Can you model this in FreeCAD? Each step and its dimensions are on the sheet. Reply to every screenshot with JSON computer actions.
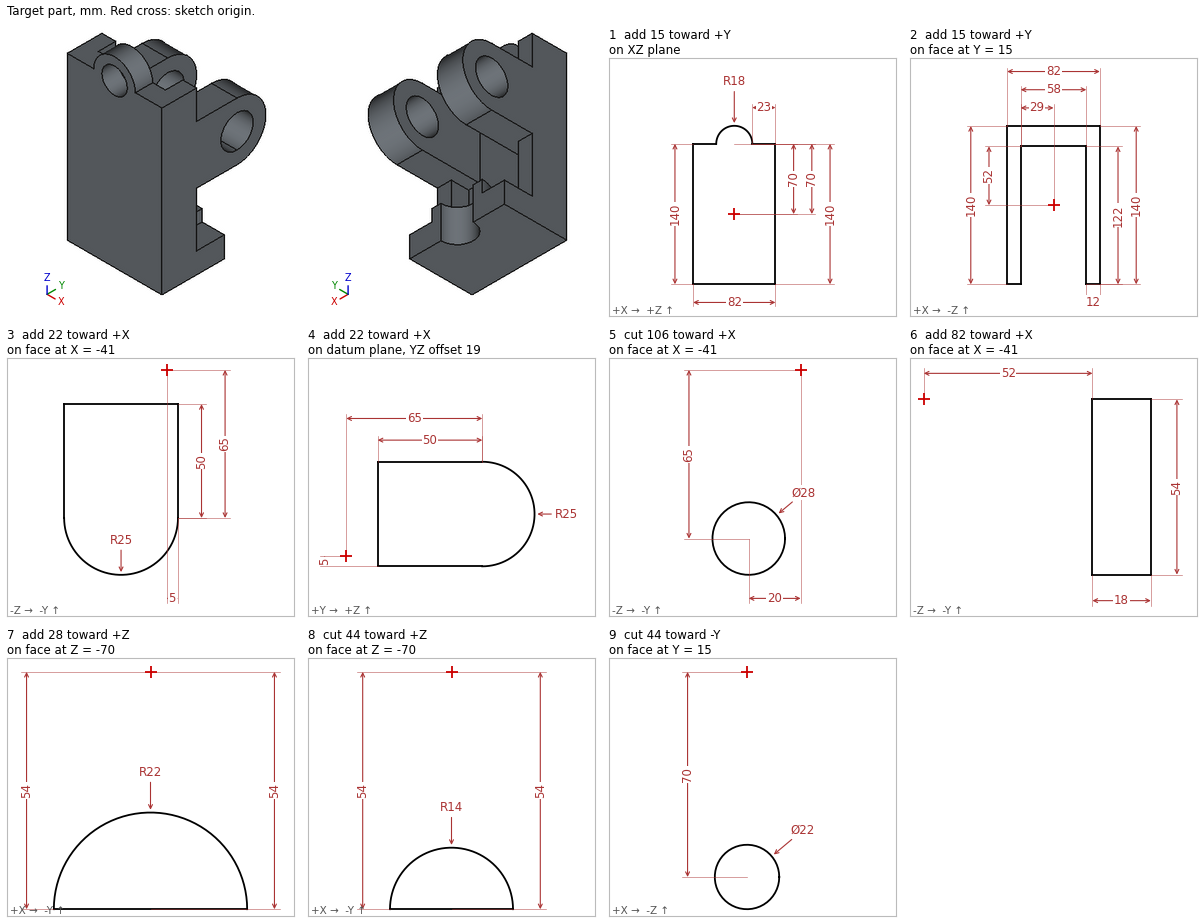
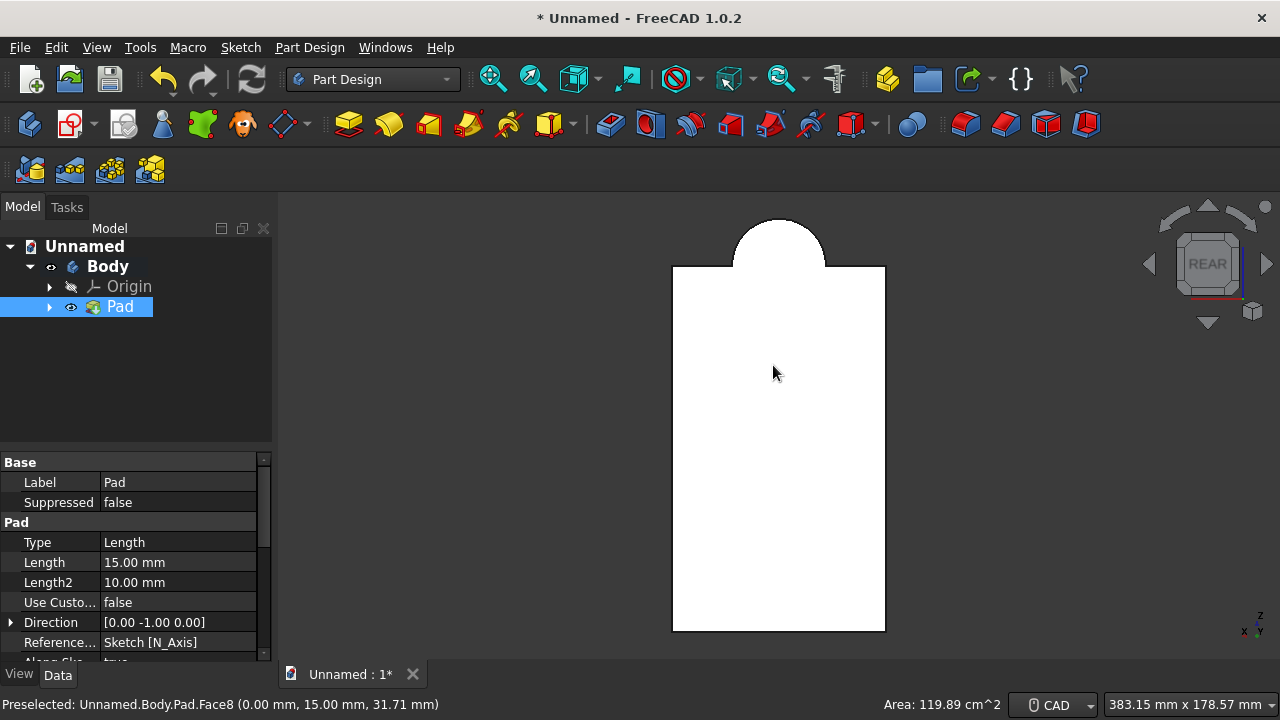
{"action": "left_click", "coordinate": [70, 124]}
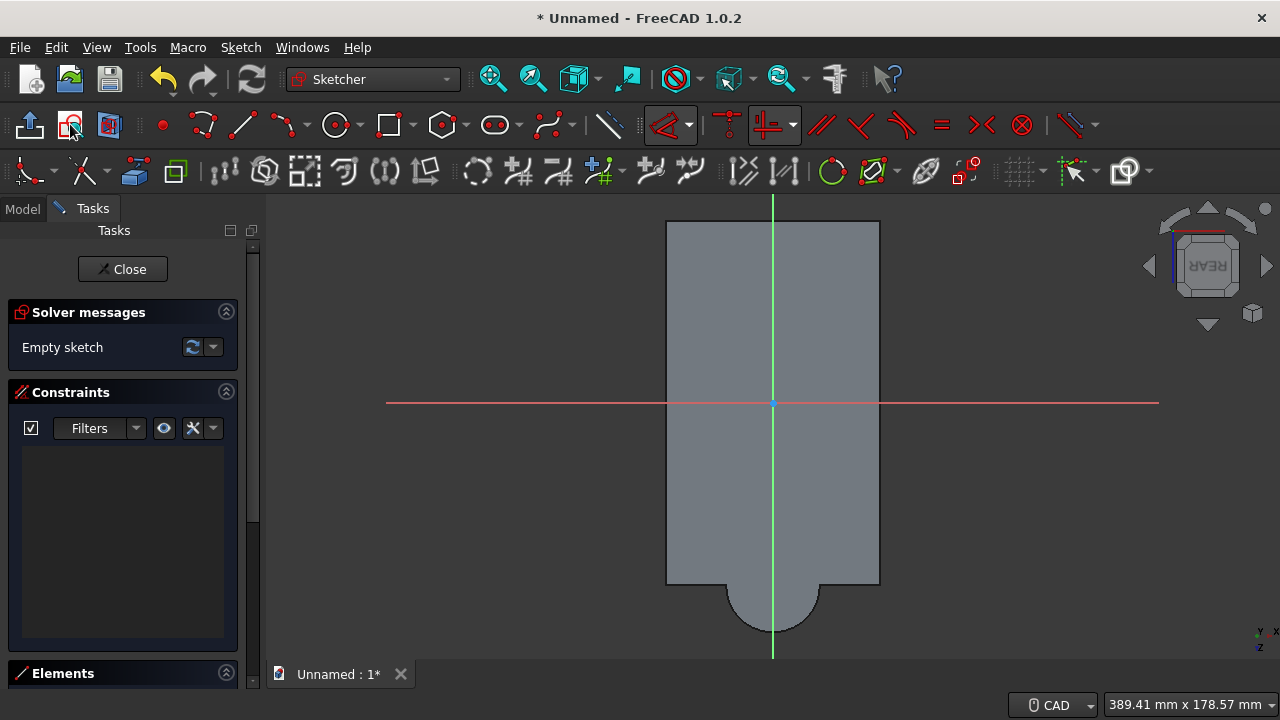
{"action": "scroll", "coordinate": [395, 532], "scroll_direction": "down", "scroll_amount": 1}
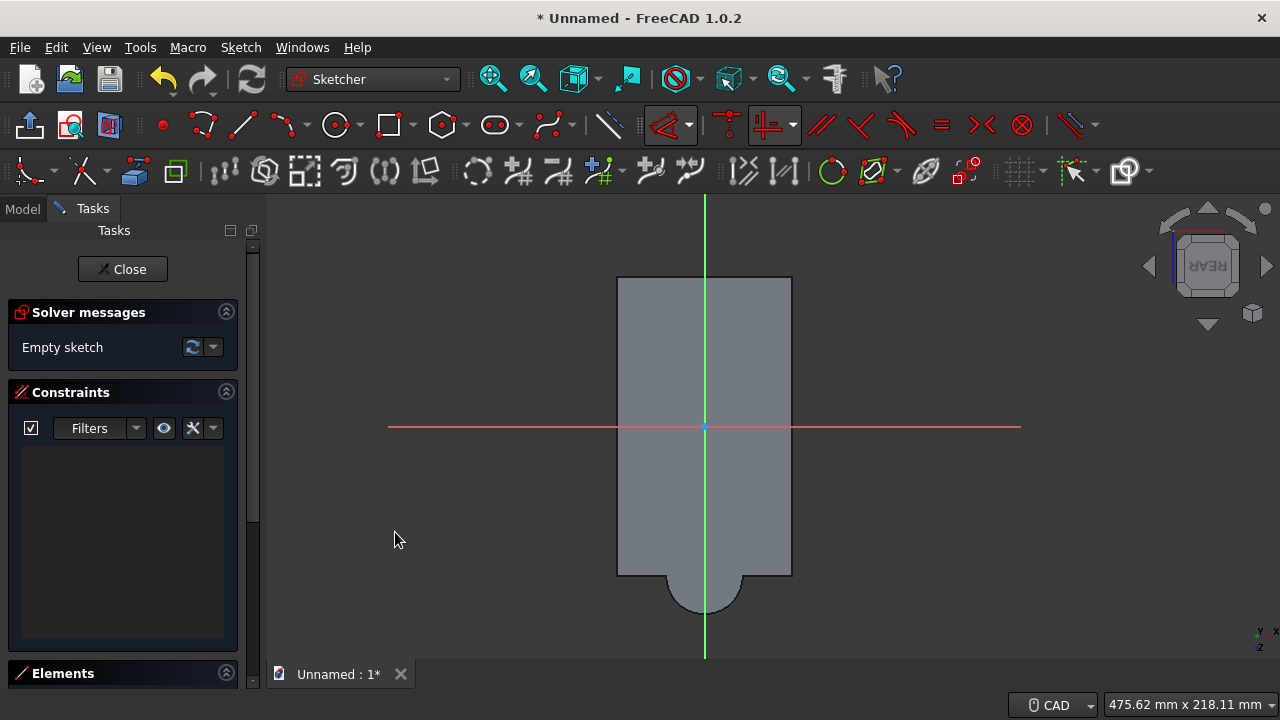
{"action": "key", "text": "g m"}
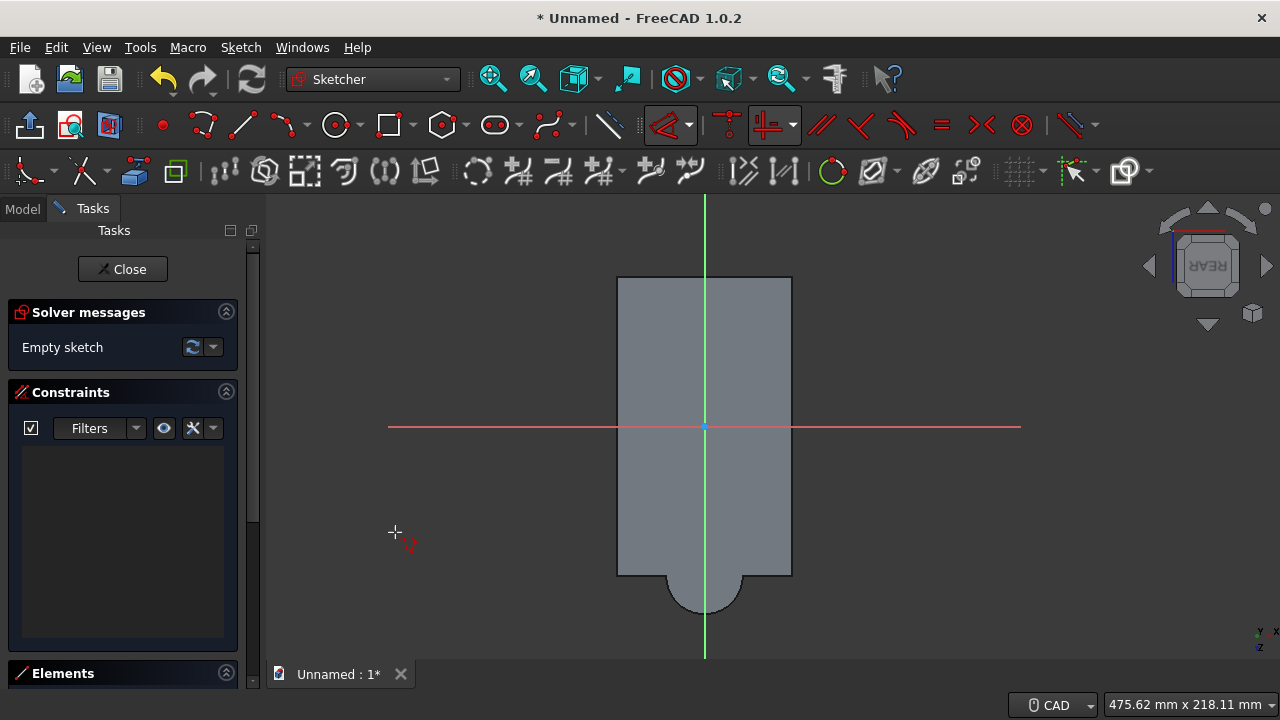
{"action": "left_click", "coordinate": [643, 316]}
{"action": "left_click", "coordinate": [766, 316]}
{"action": "left_click", "coordinate": [766, 576]}
{"action": "left_click", "coordinate": [792, 576]}
{"action": "left_click", "coordinate": [792, 277]}
{"action": "left_click", "coordinate": [617, 277]}
{"action": "left_click", "coordinate": [617, 576]}
{"action": "left_click", "coordinate": [643, 576]}
{"action": "left_click", "coordinate": [643, 317]}
{"action": "key", "text": "Escape"}
{"action": "key", "text": "Escape"}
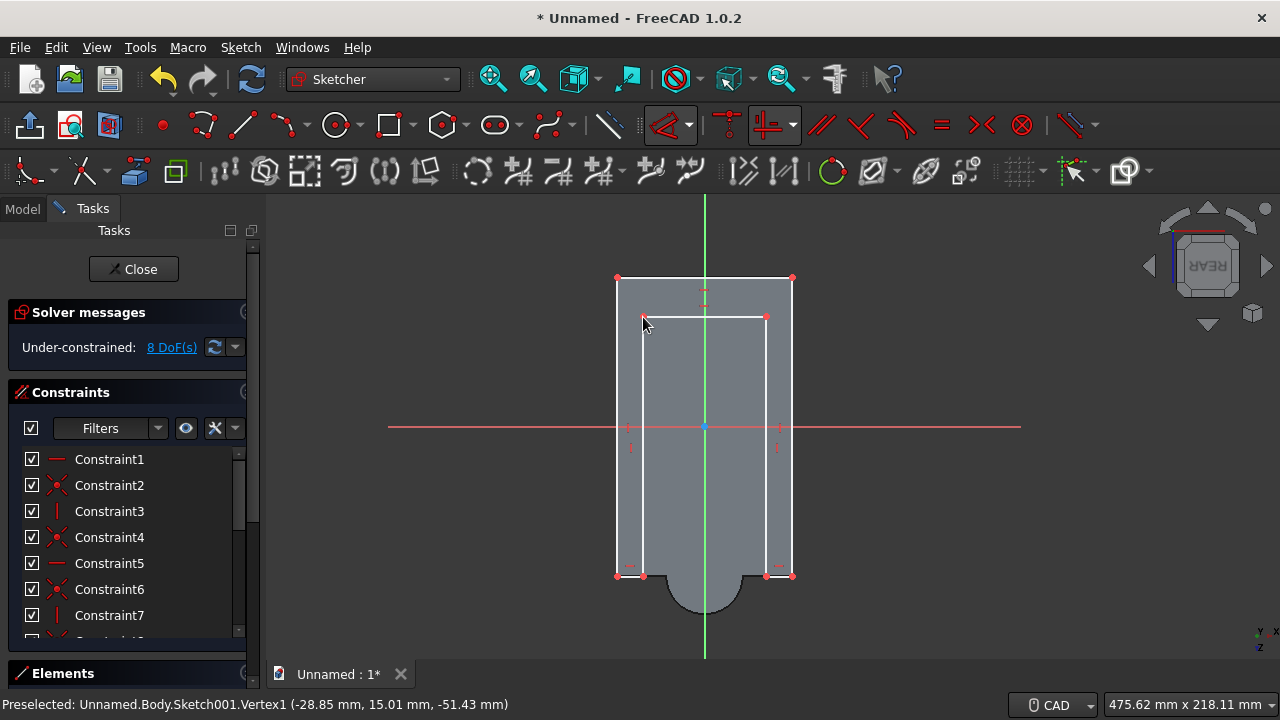
{"action": "left_click", "coordinate": [680, 317]}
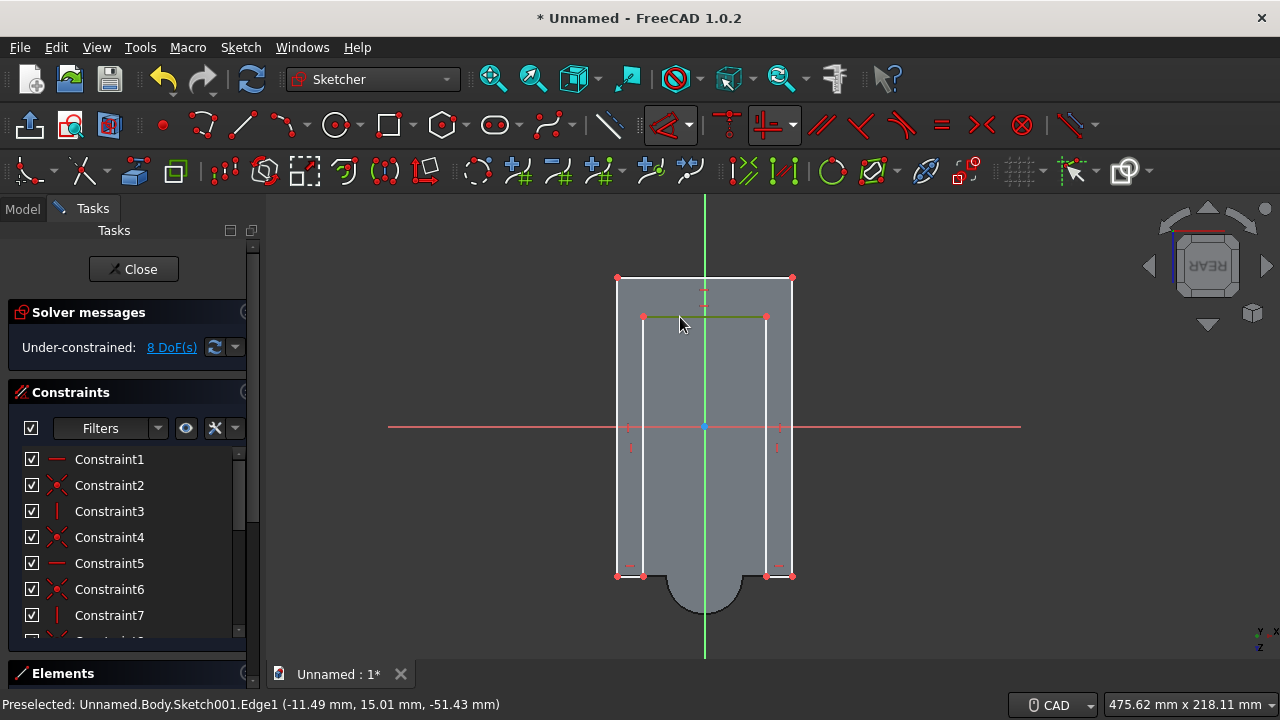
{"action": "key", "text": "l"}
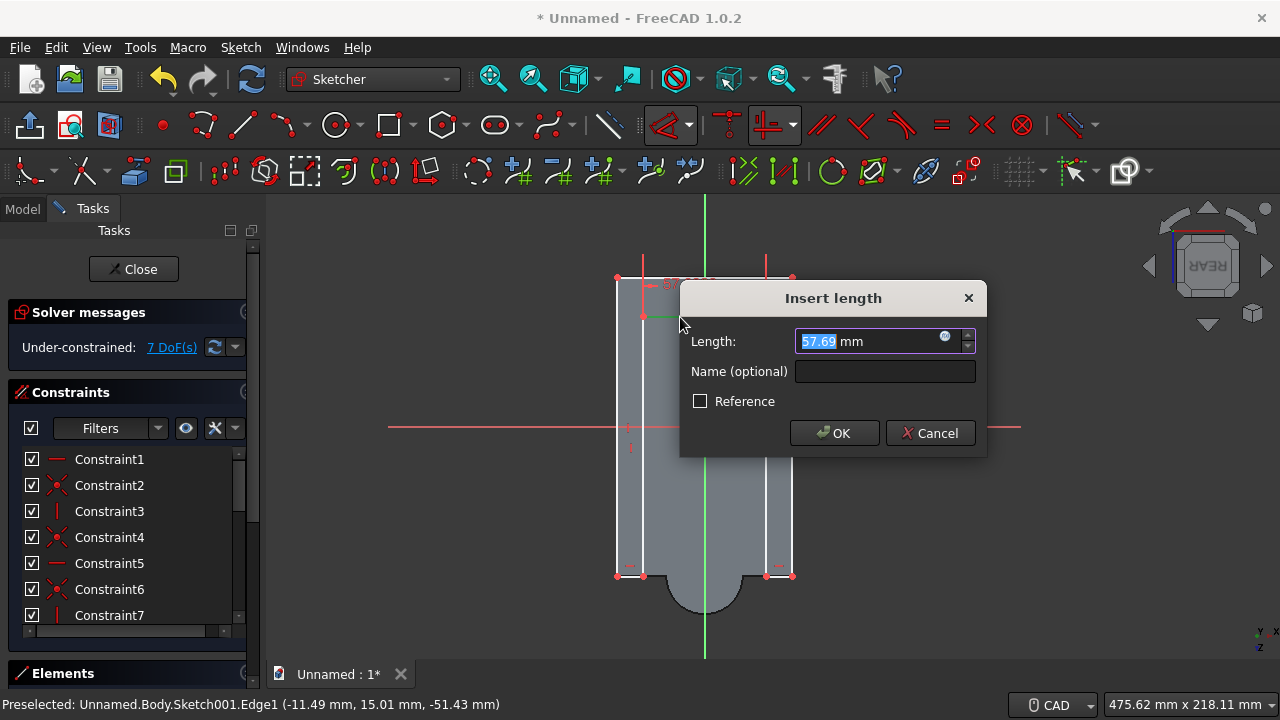
{"action": "type", "text": "58"}
{"action": "key", "text": "Return"}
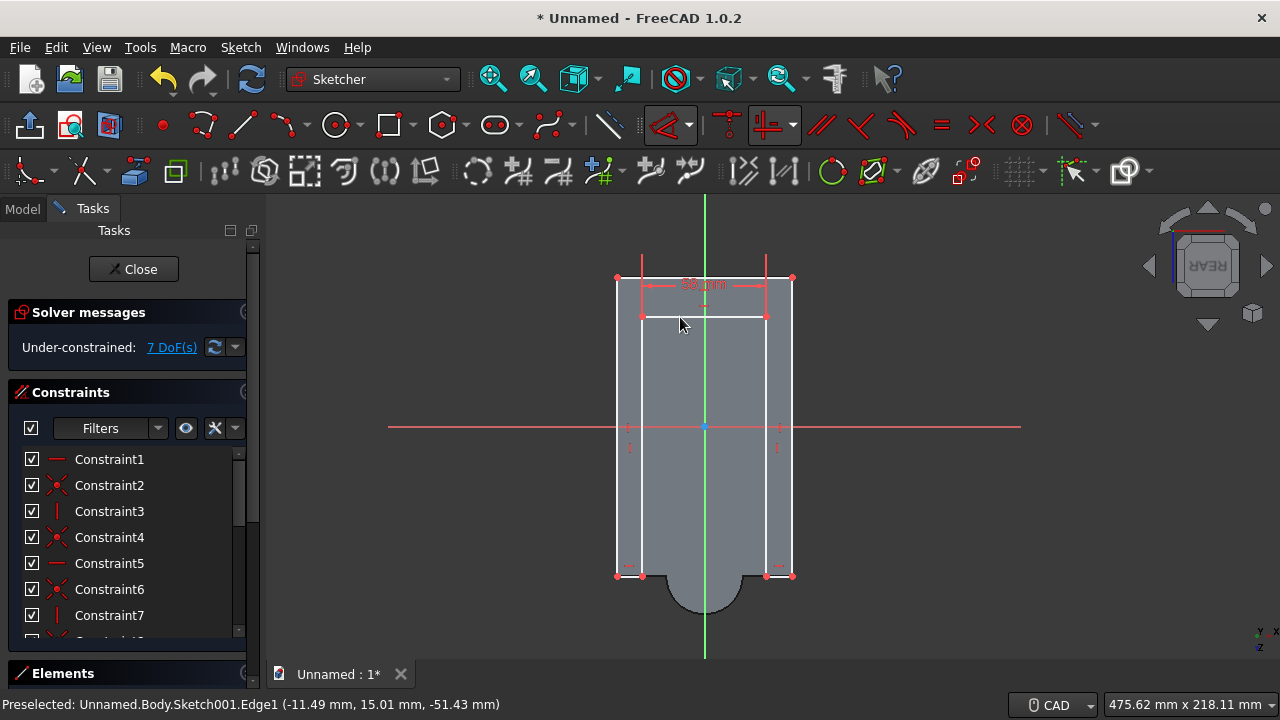
{"action": "scroll", "coordinate": [776, 577], "scroll_direction": "up", "scroll_amount": 3}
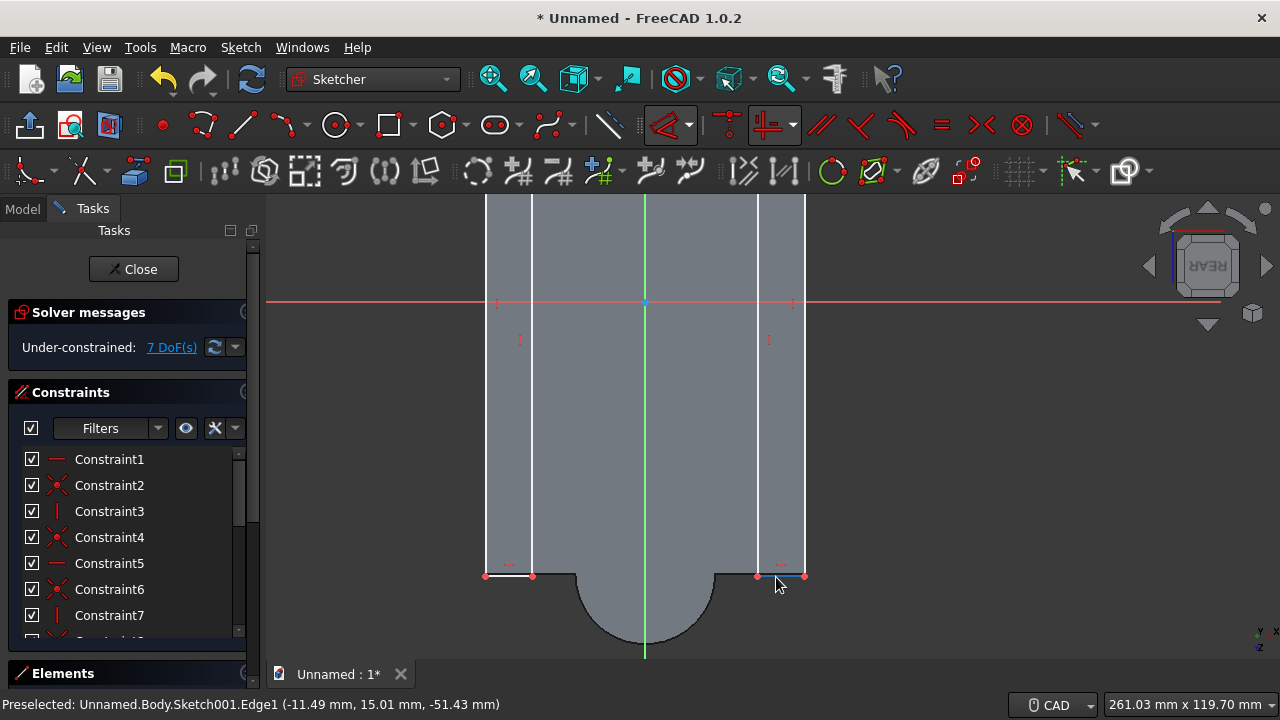
{"action": "left_click", "coordinate": [776, 576]}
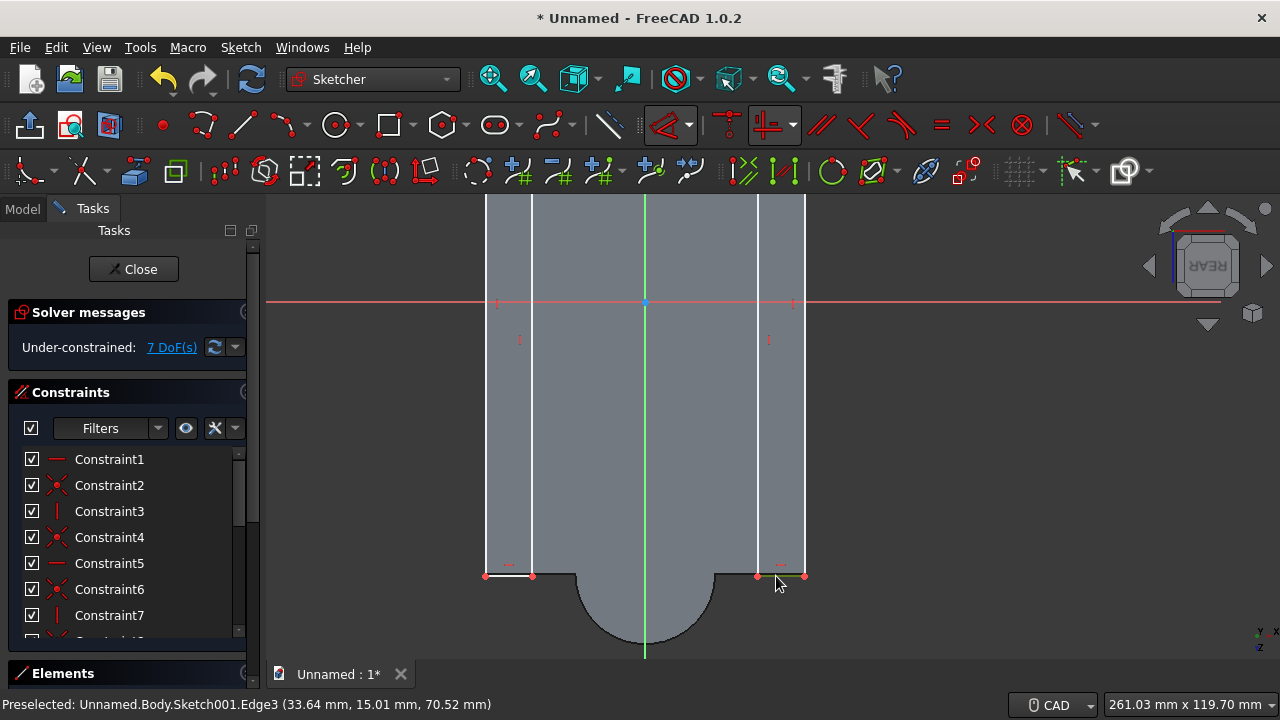
{"action": "key", "text": "l"}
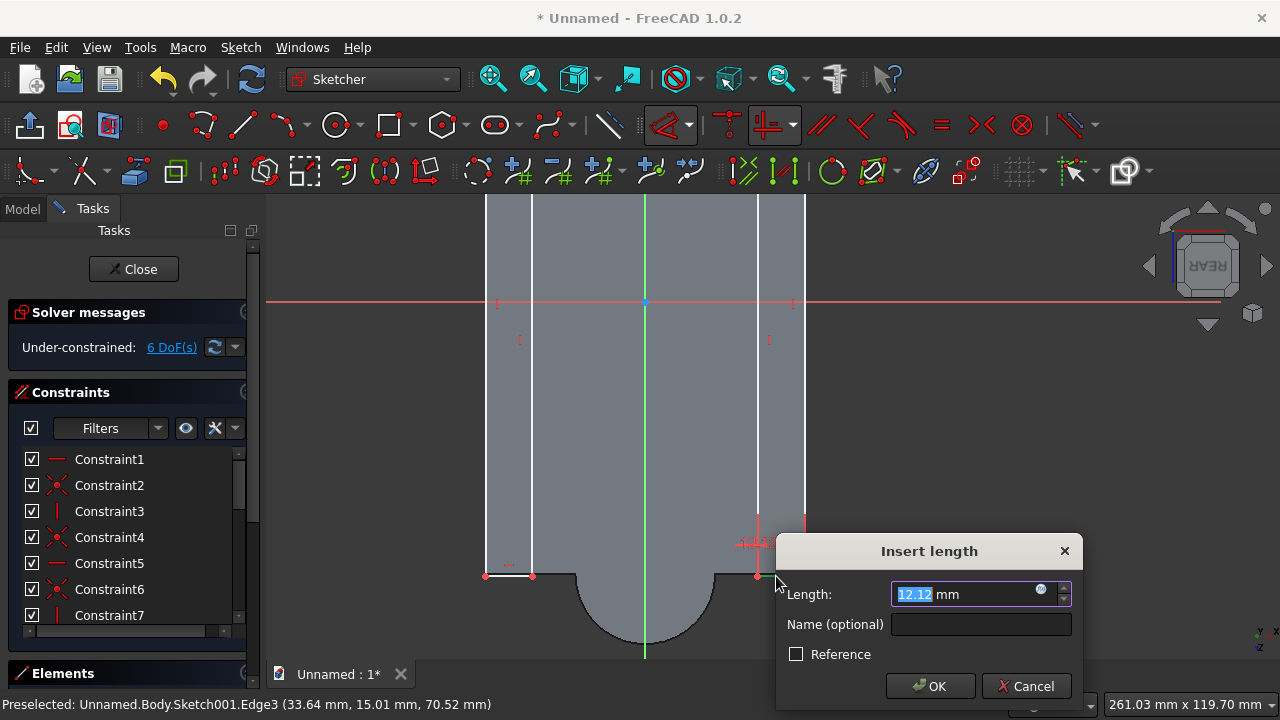
{"action": "type", "text": "12"}
{"action": "key", "text": "Return"}